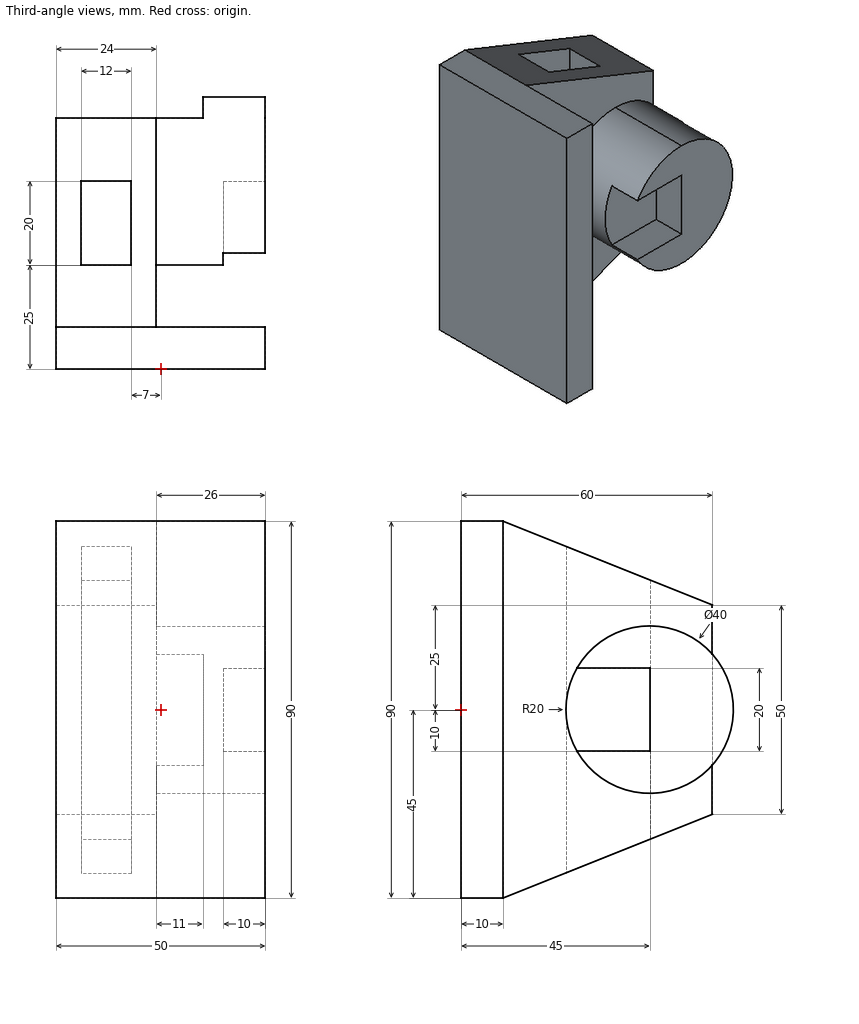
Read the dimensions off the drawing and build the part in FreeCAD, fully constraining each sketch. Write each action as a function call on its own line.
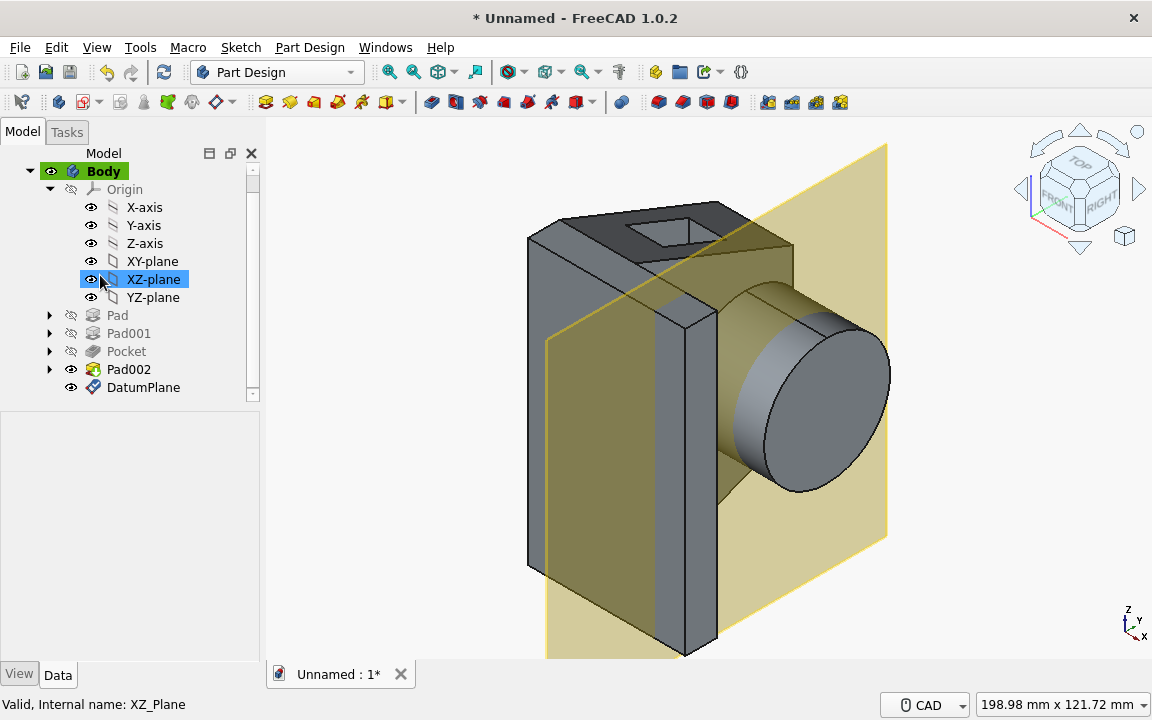
click(116, 387)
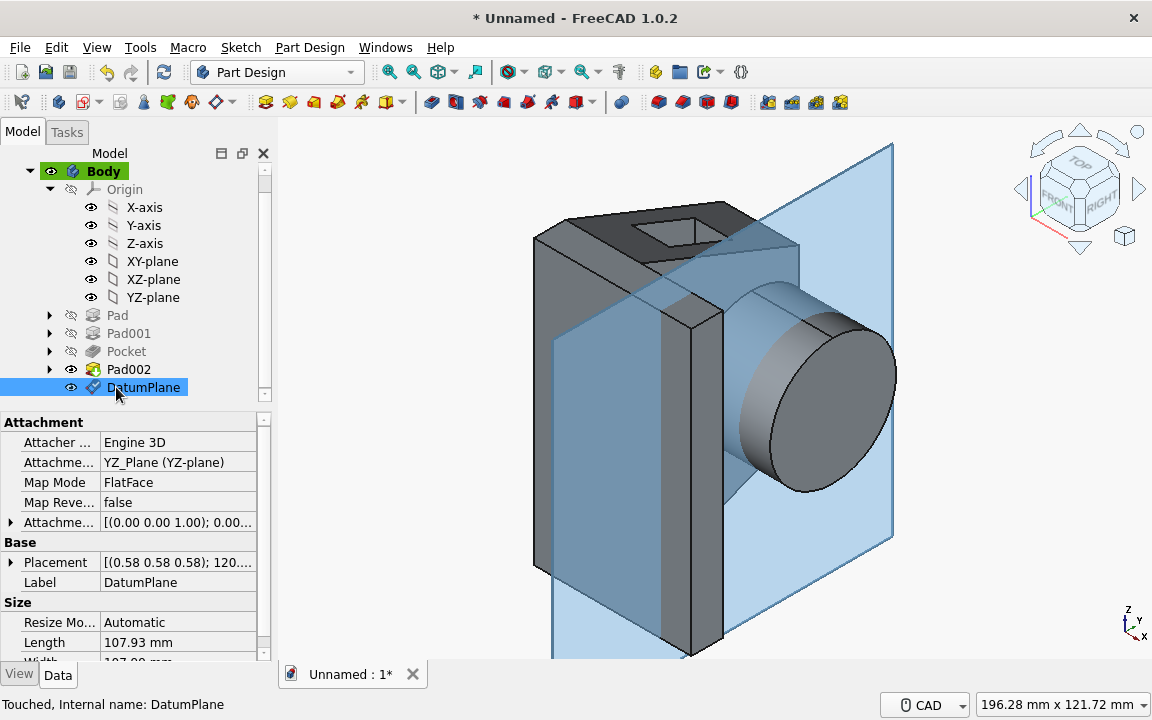
click(84, 102)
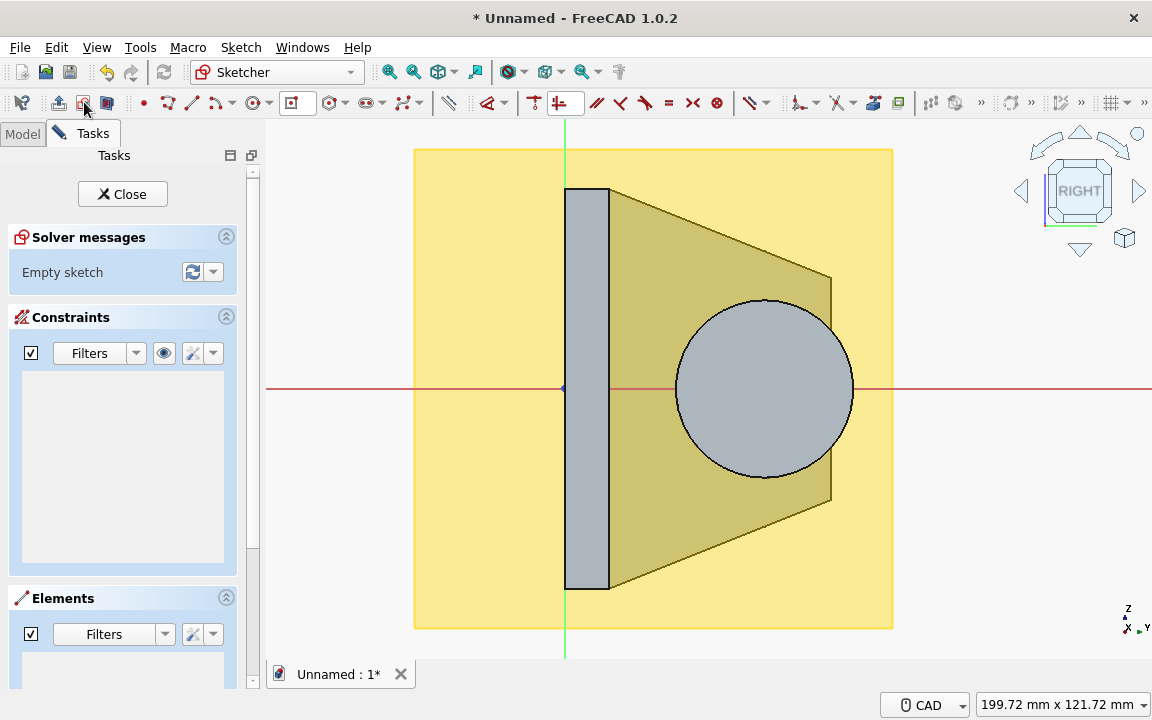
click(108, 104)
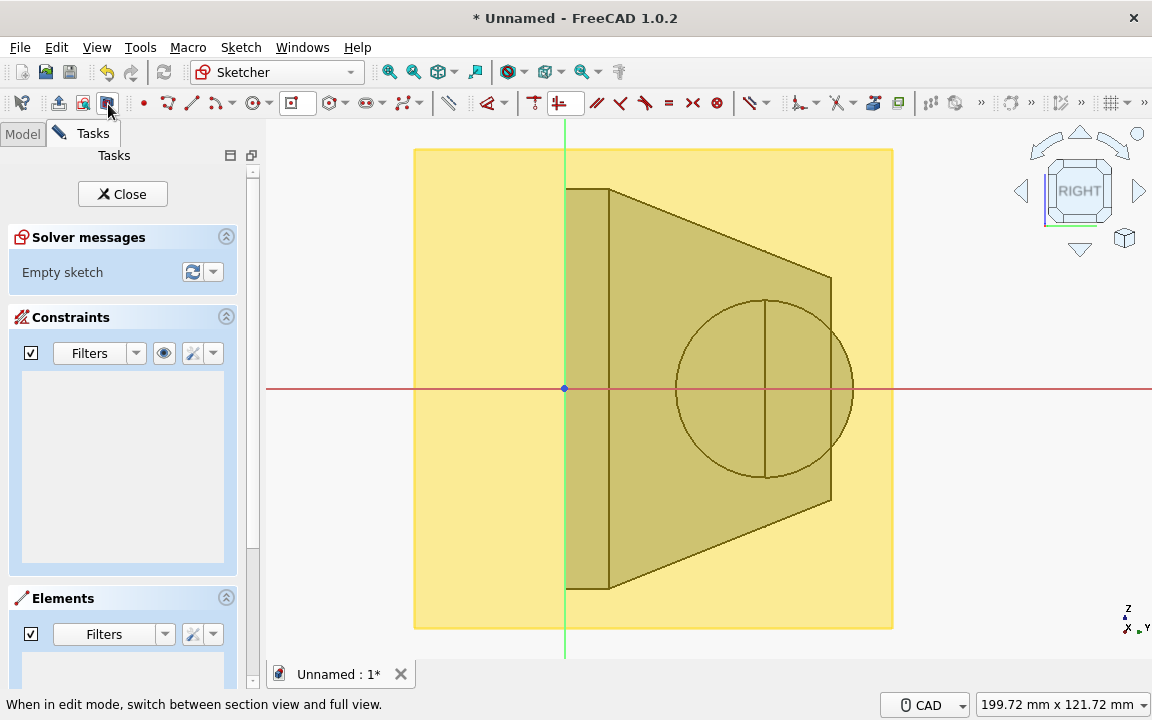
scroll(685, 389, up, 4)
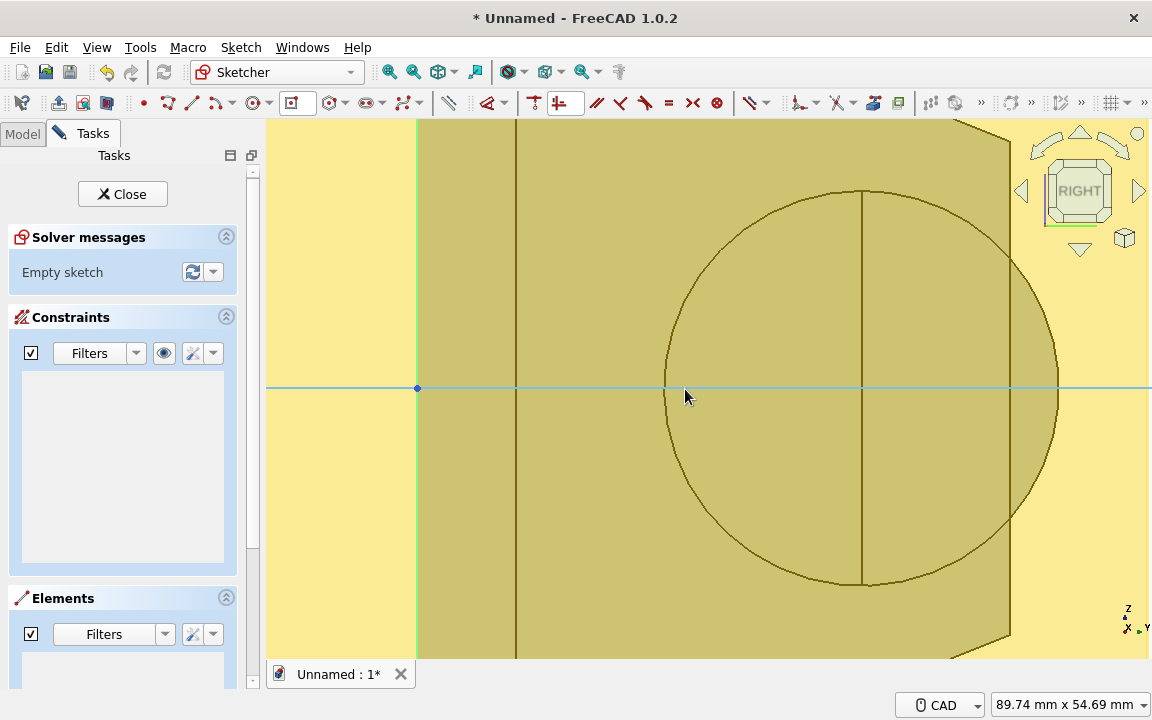
click(168, 104)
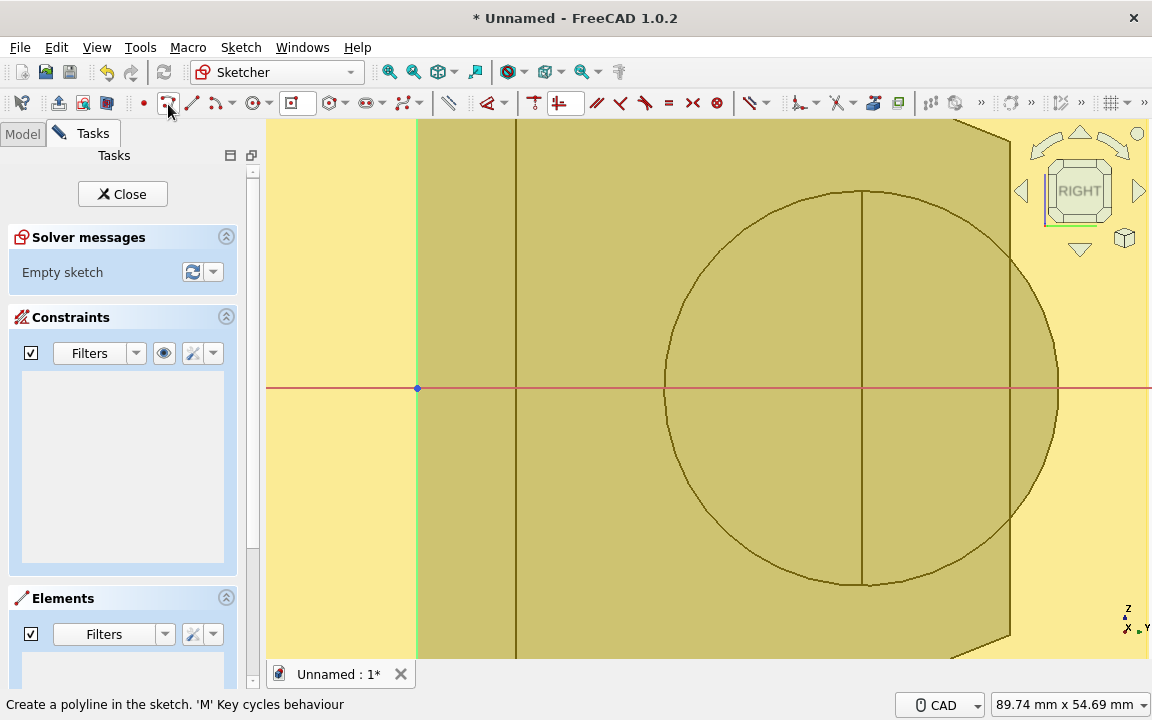
click(691, 487)
click(862, 487)
click(862, 290)
click(691, 290)
right_click(691, 290)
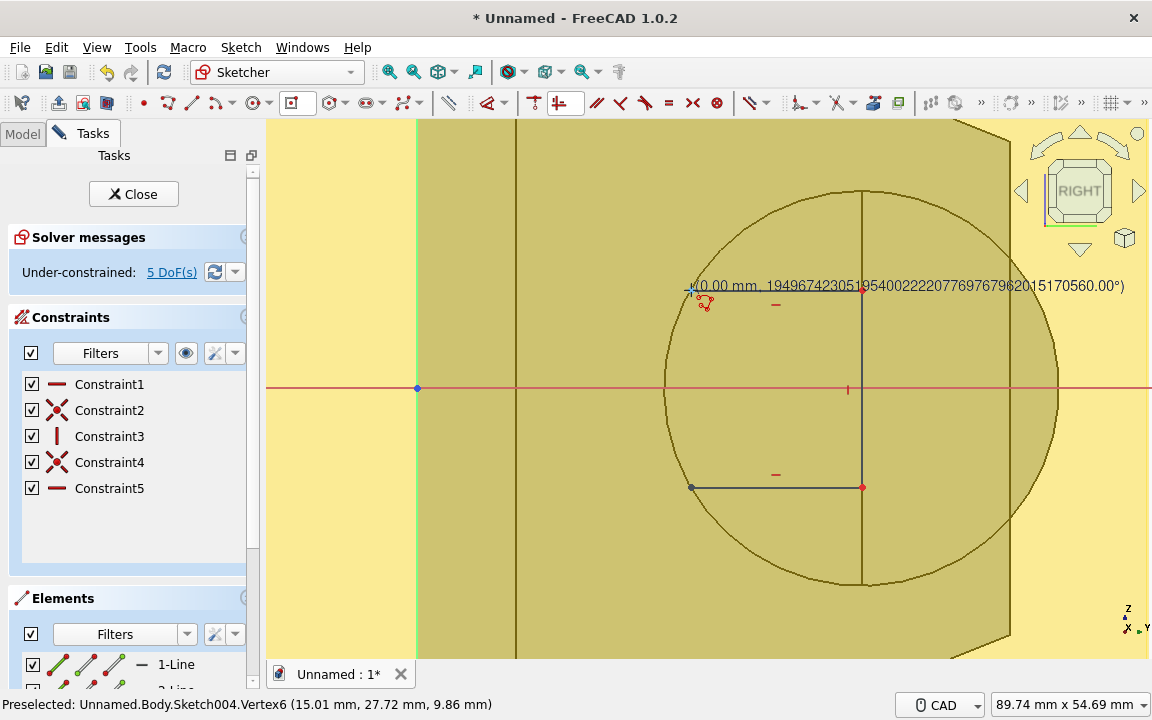
key(g)
key(3)
key(a)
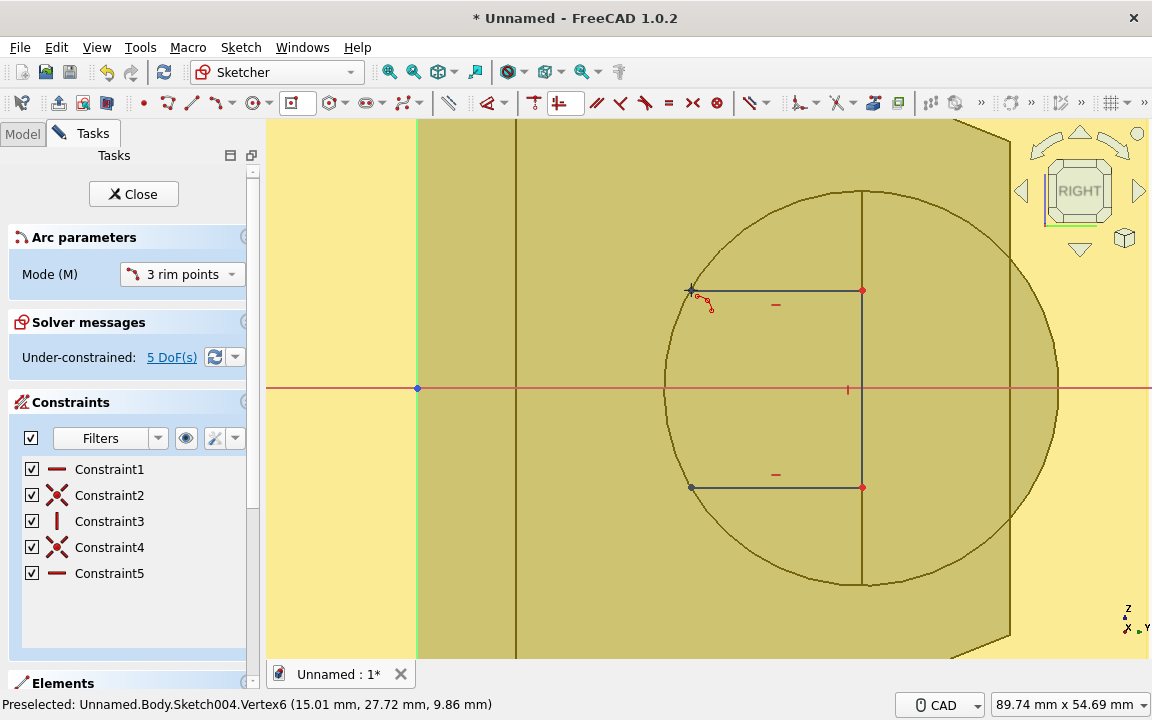
click(691, 291)
click(691, 488)
click(665, 368)
key(Escape)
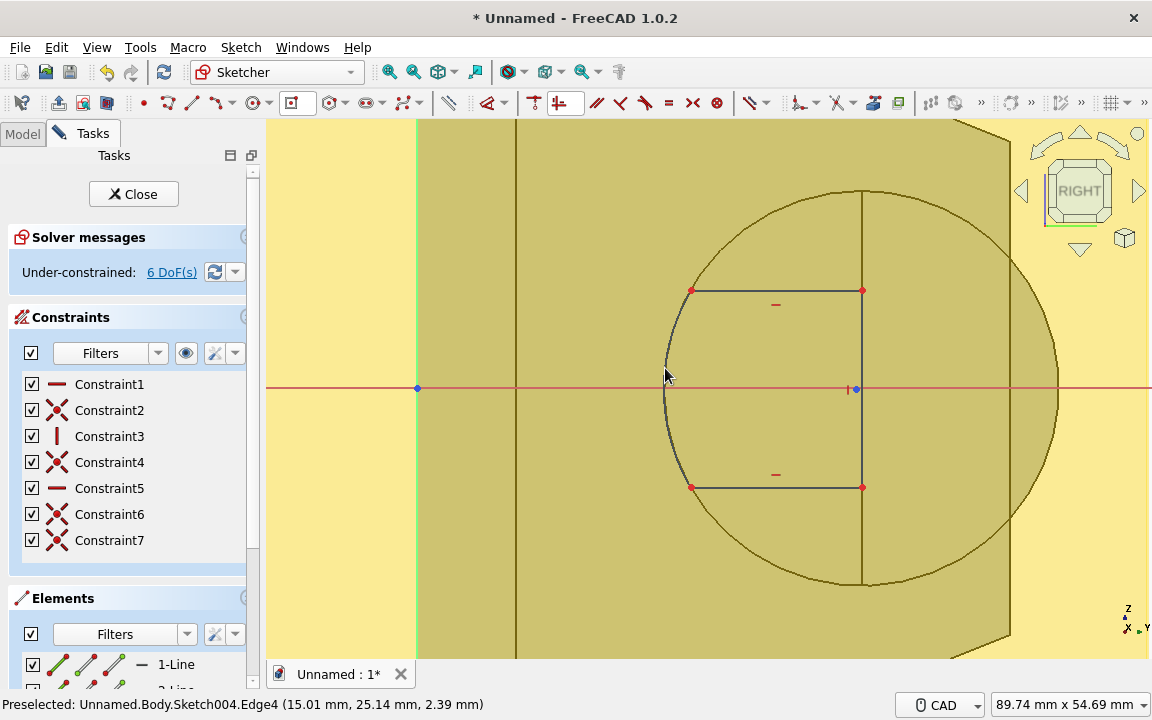
click(857, 389)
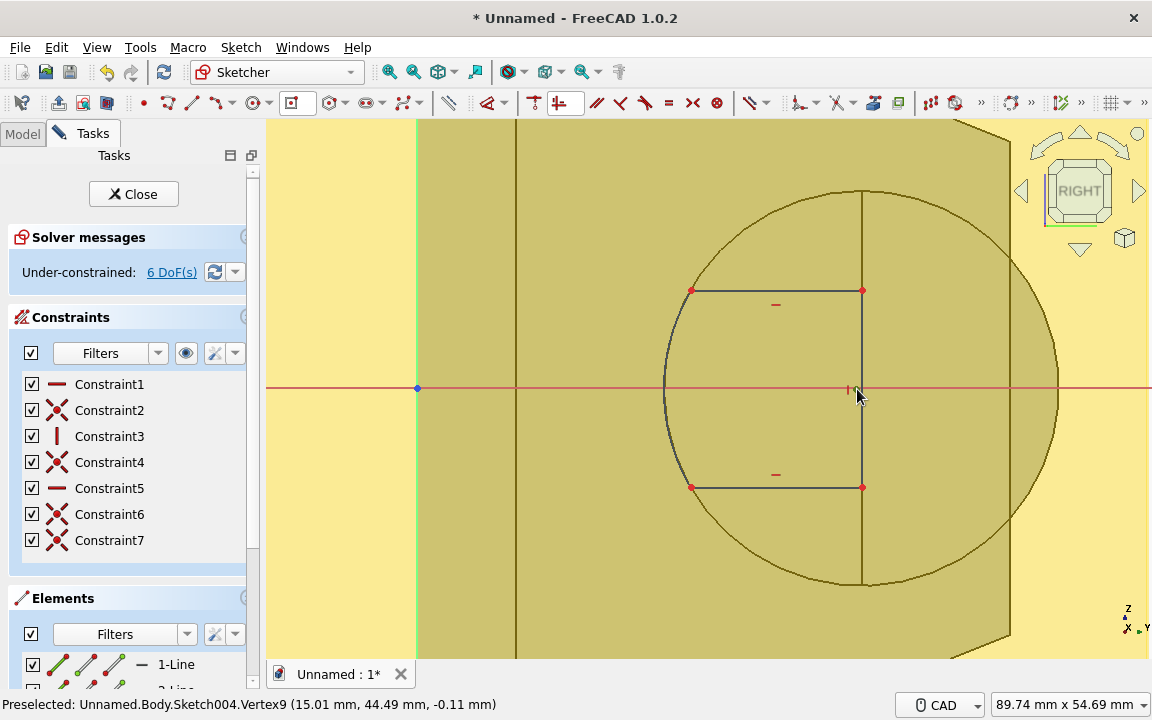
click(344, 388)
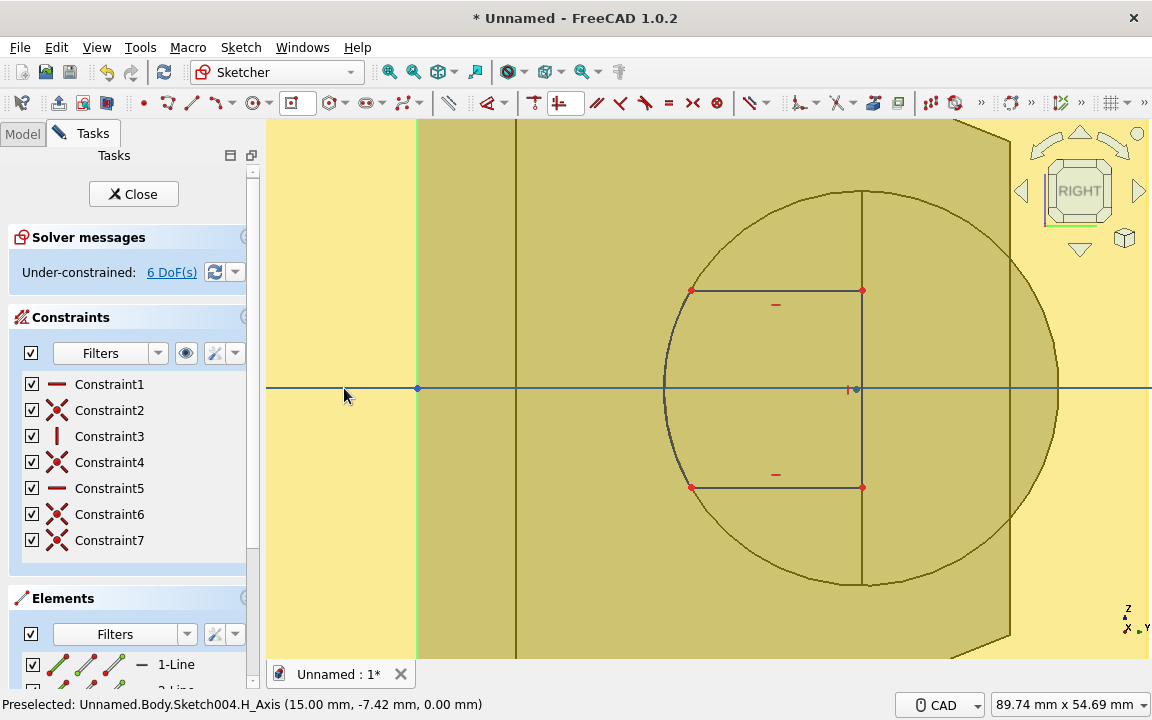
click(534, 104)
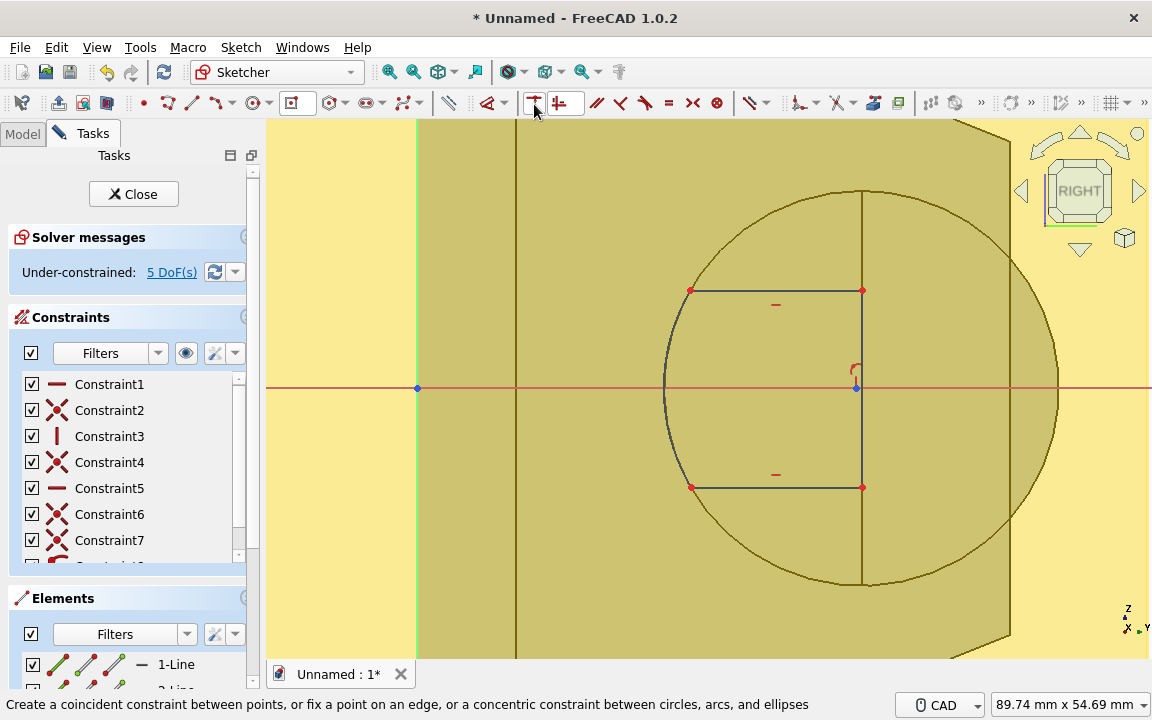
click(488, 104)